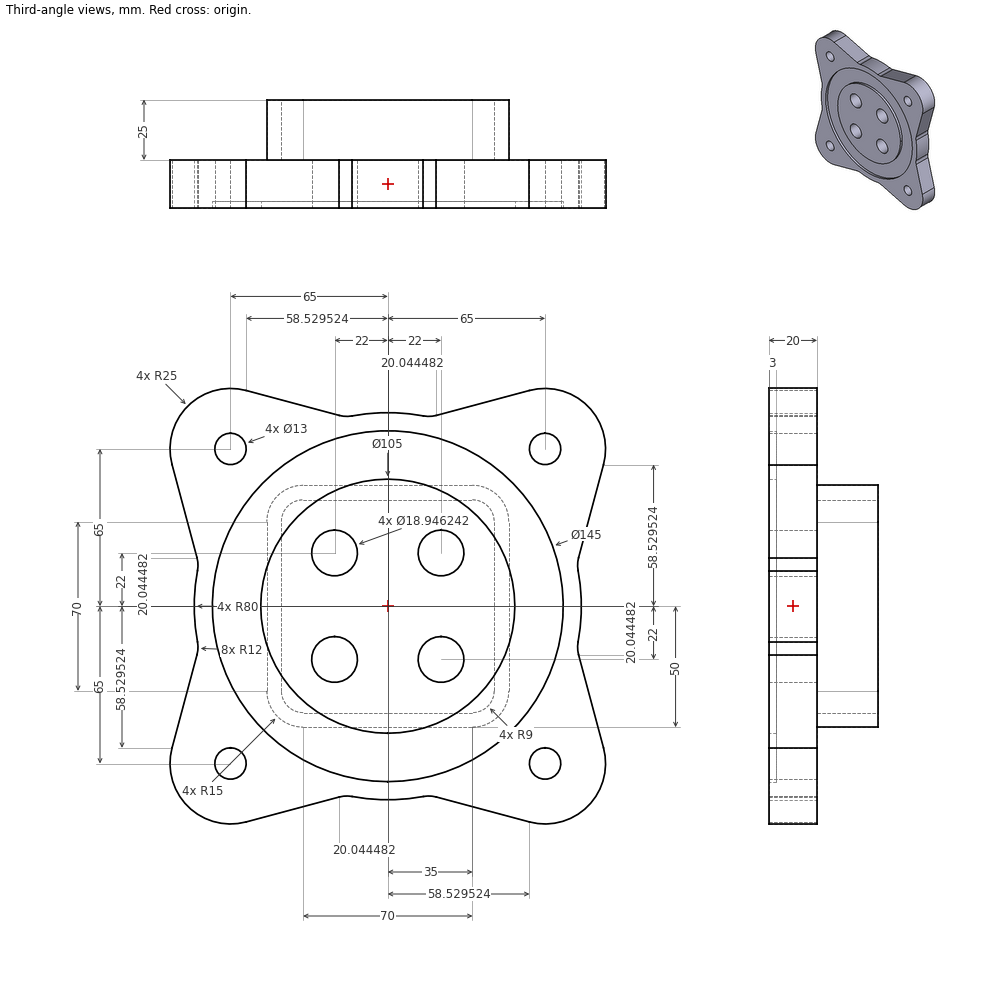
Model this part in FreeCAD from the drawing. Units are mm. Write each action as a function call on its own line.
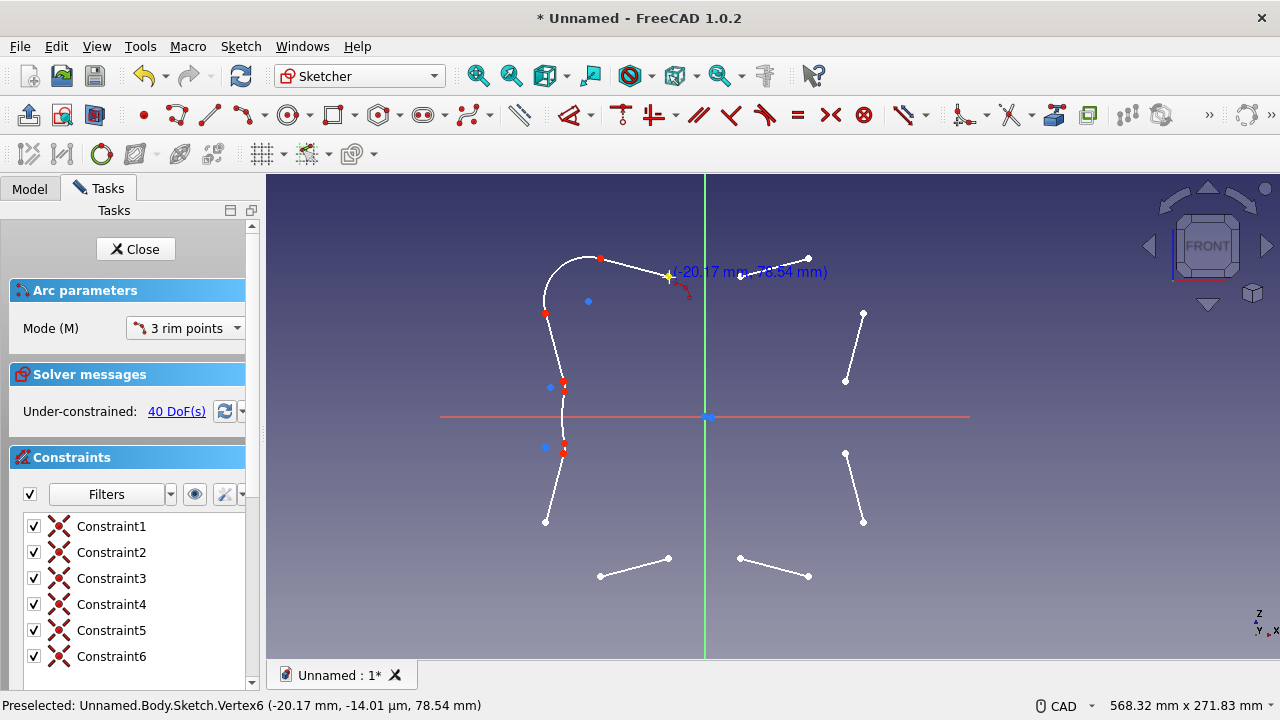
scroll(679, 277, up, 3)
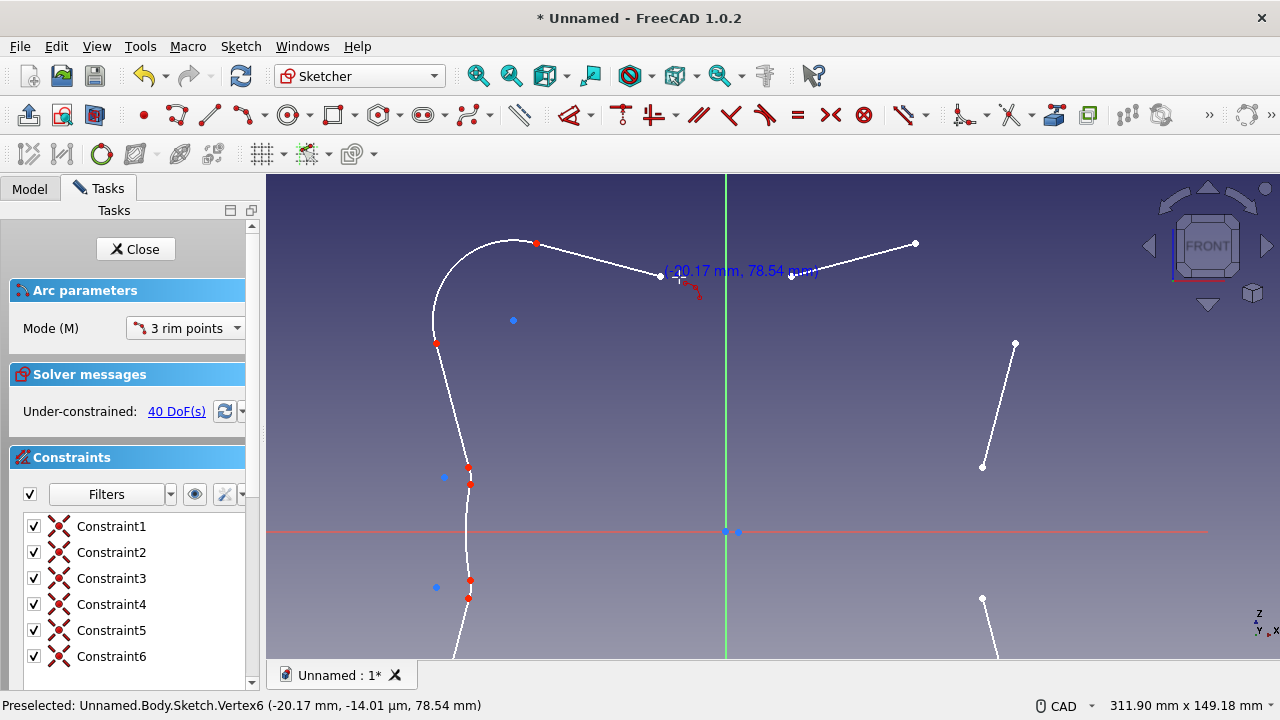
click(678, 276)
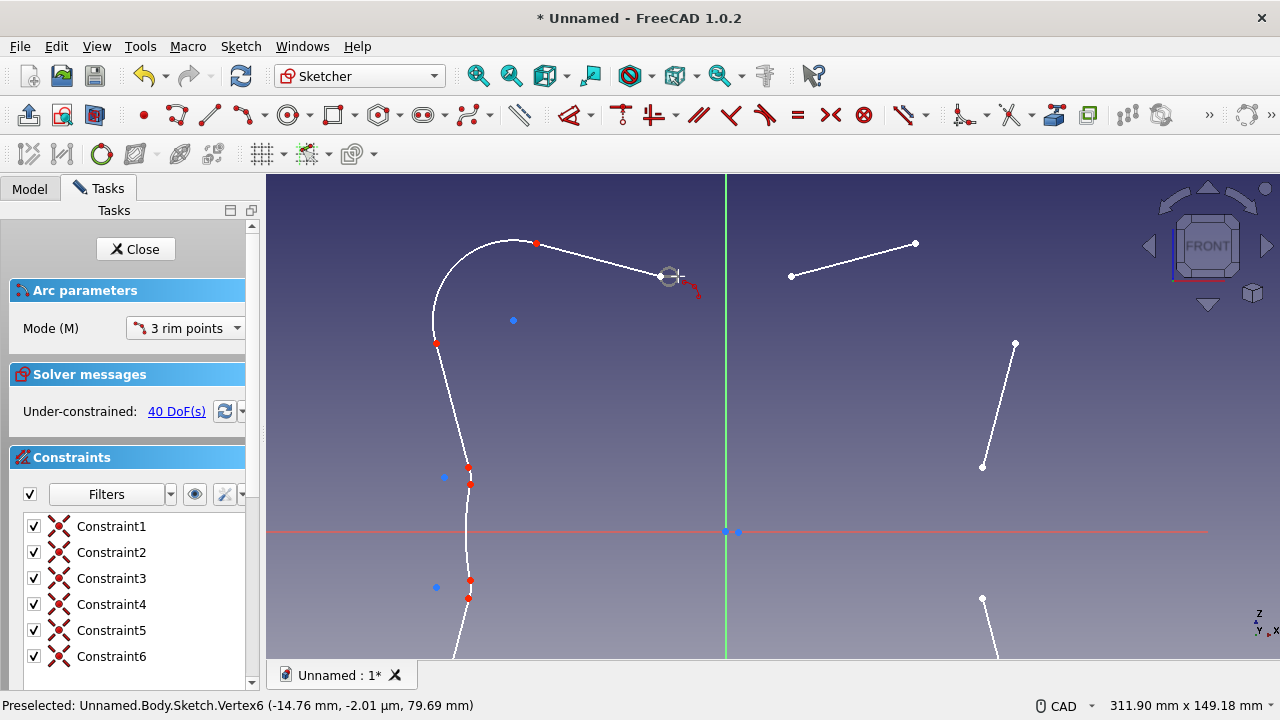
scroll(669, 277, up, 14)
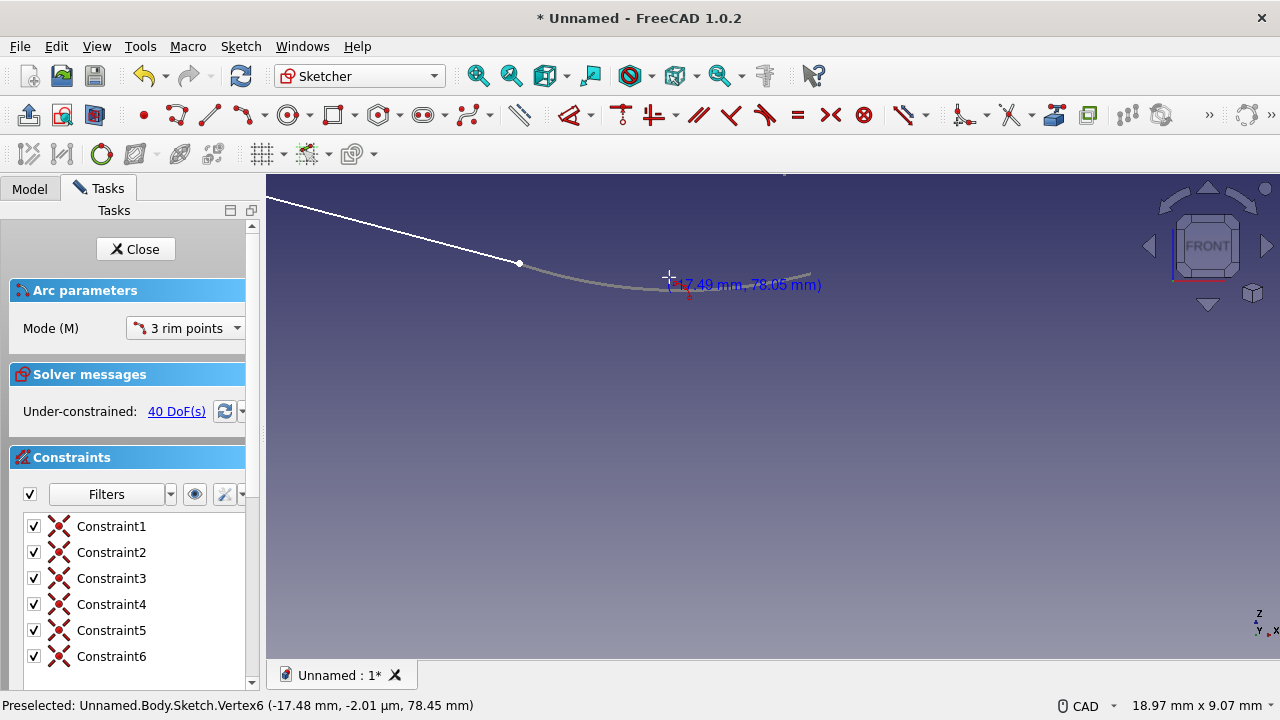
click(668, 270)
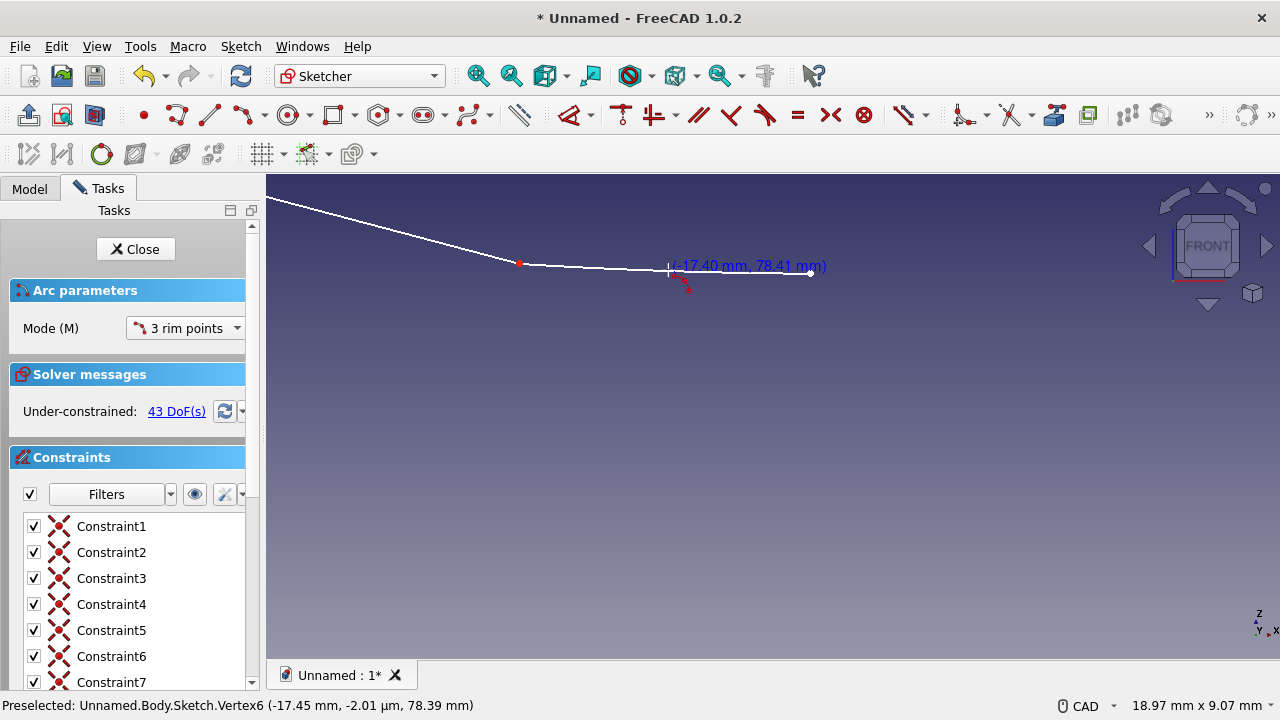
scroll(674, 277, down, 17)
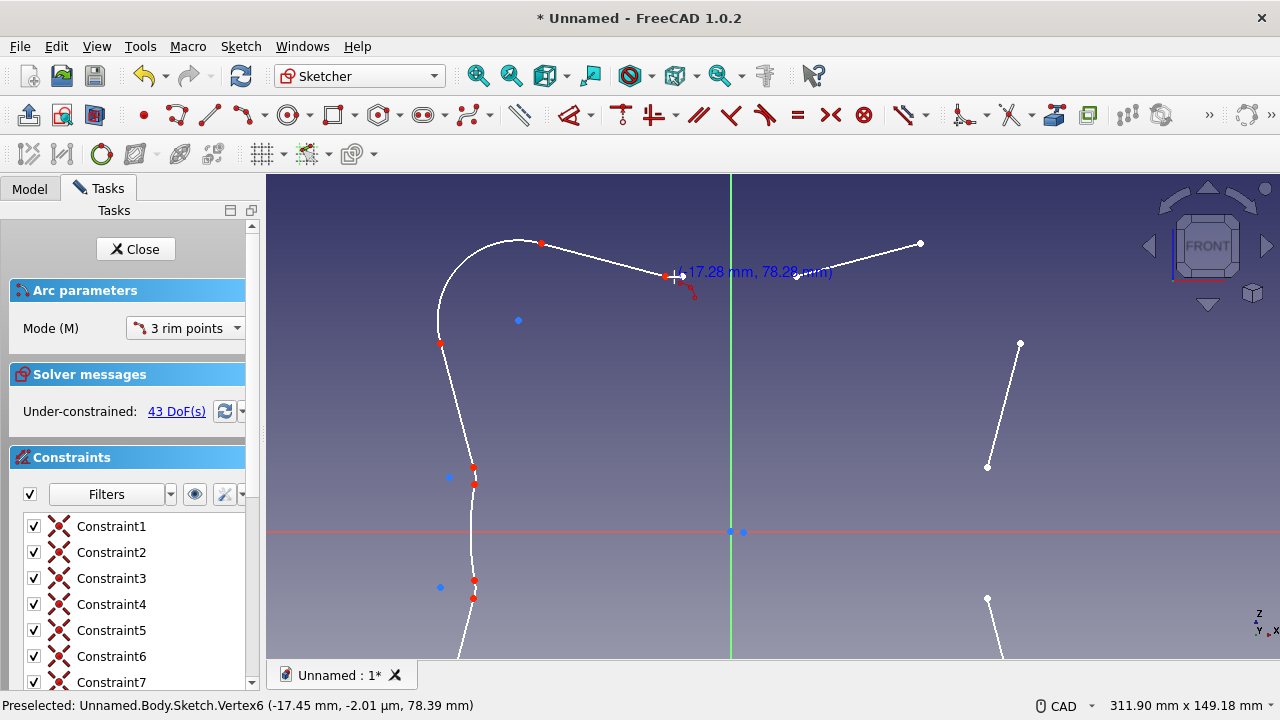
scroll(679, 277, up, 3)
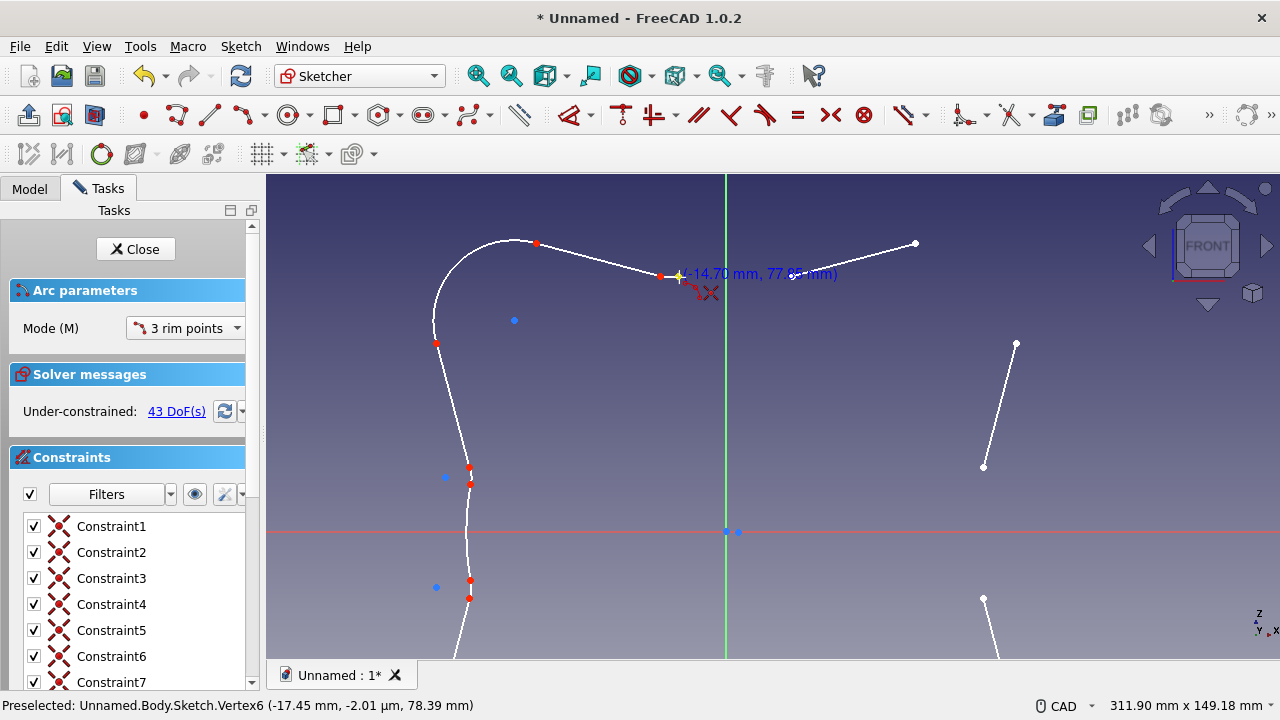
click(679, 277)
click(774, 276)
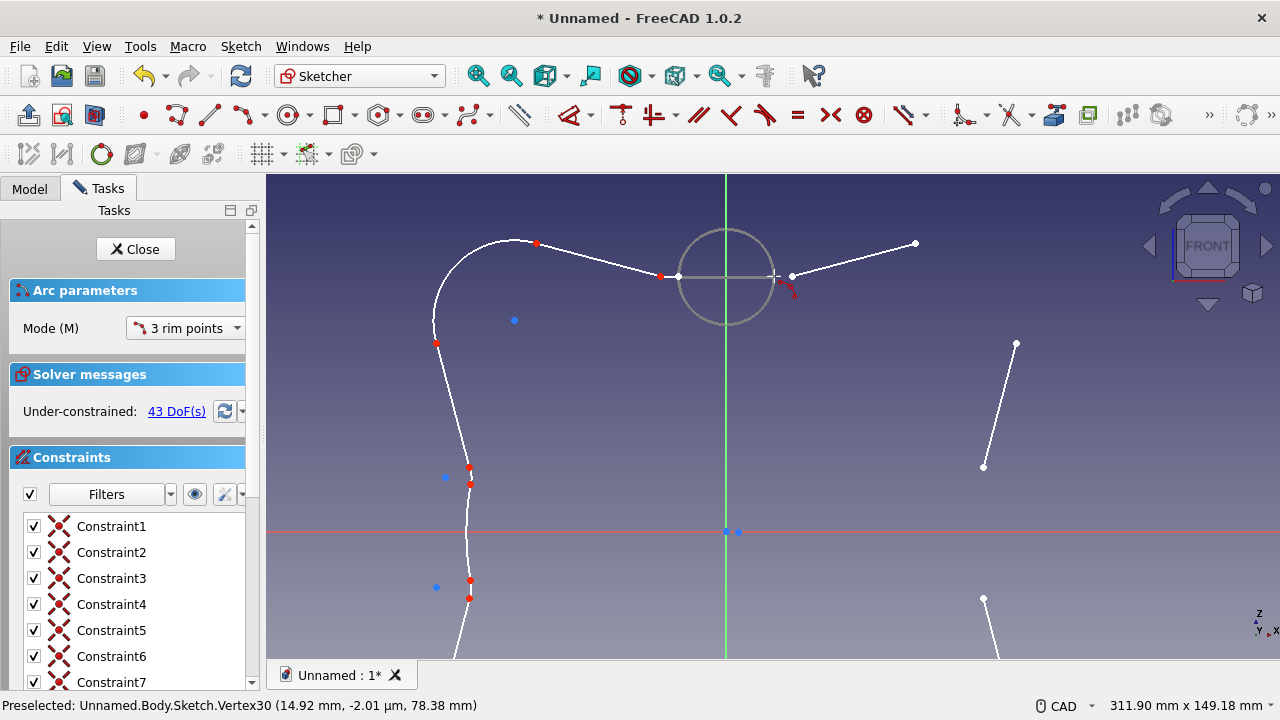
scroll(736, 272, up, 7)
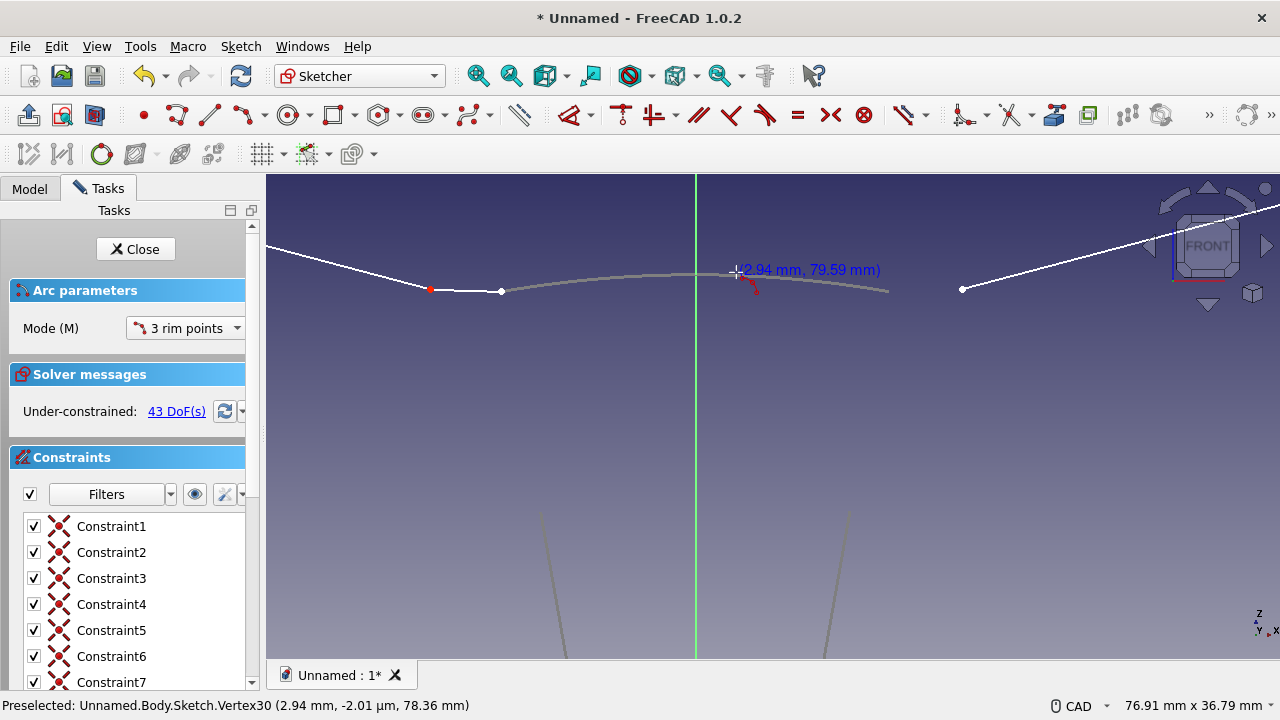
click(735, 271)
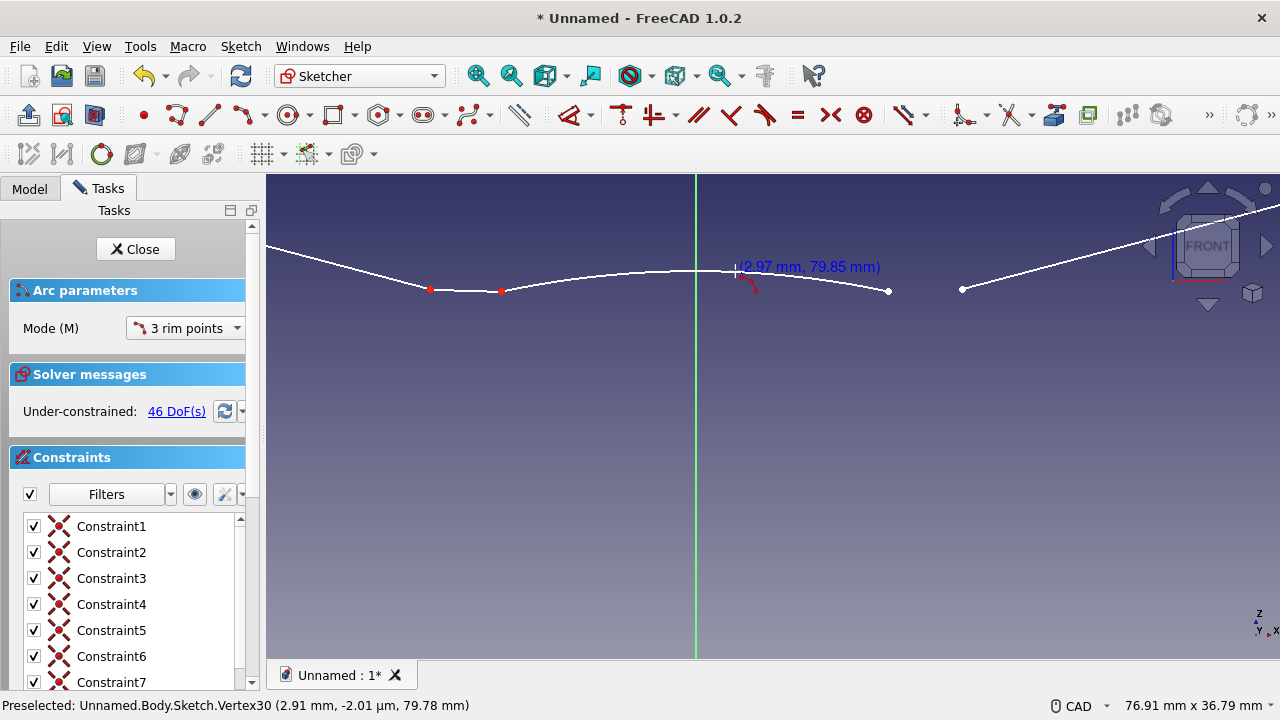
scroll(706, 274, down, 10)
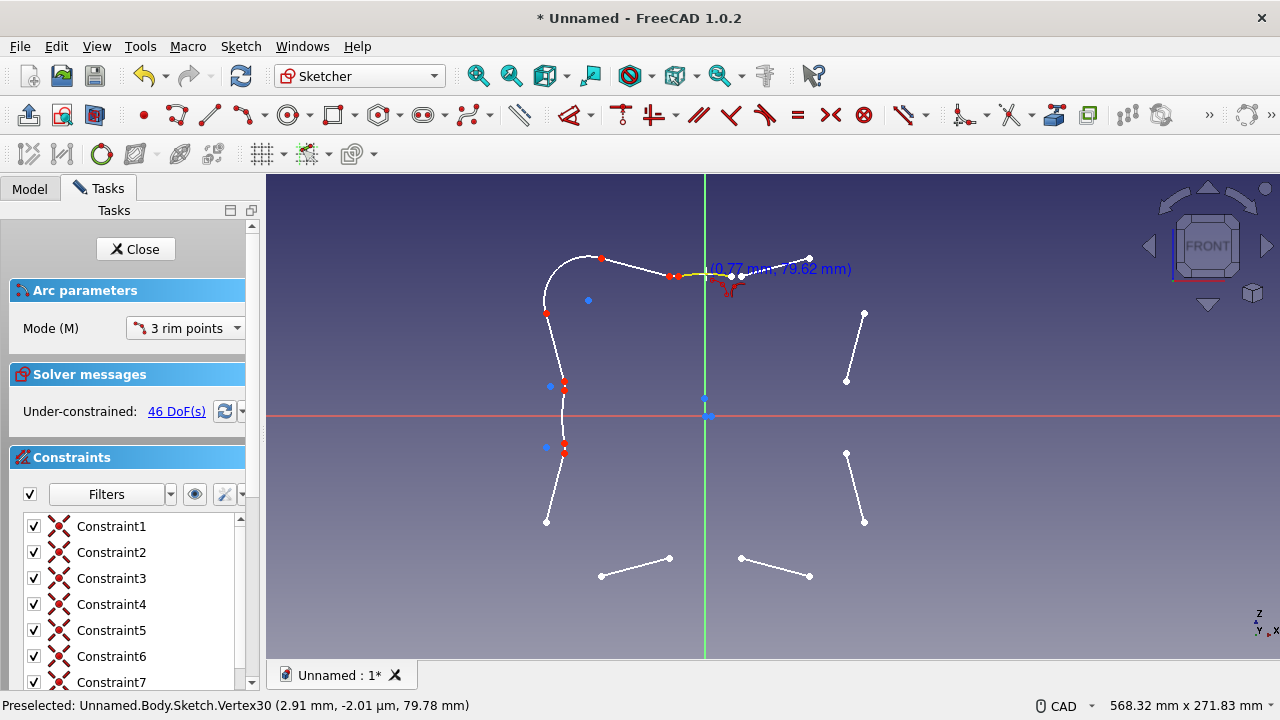
scroll(731, 276, up, 3)